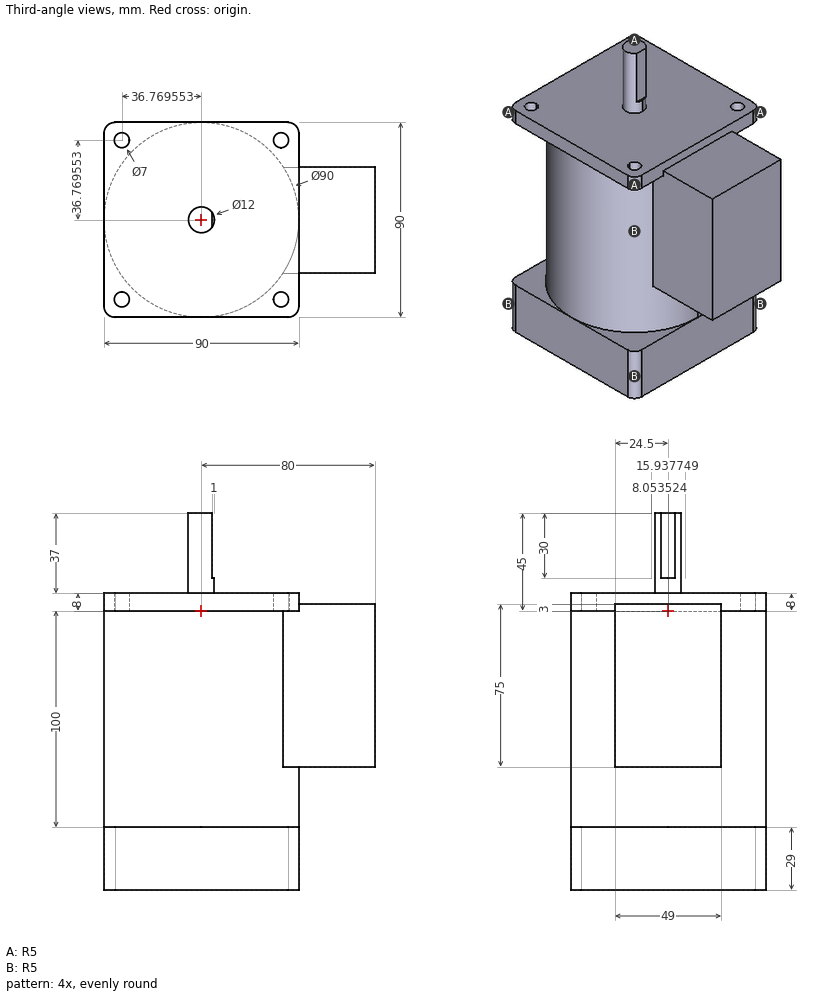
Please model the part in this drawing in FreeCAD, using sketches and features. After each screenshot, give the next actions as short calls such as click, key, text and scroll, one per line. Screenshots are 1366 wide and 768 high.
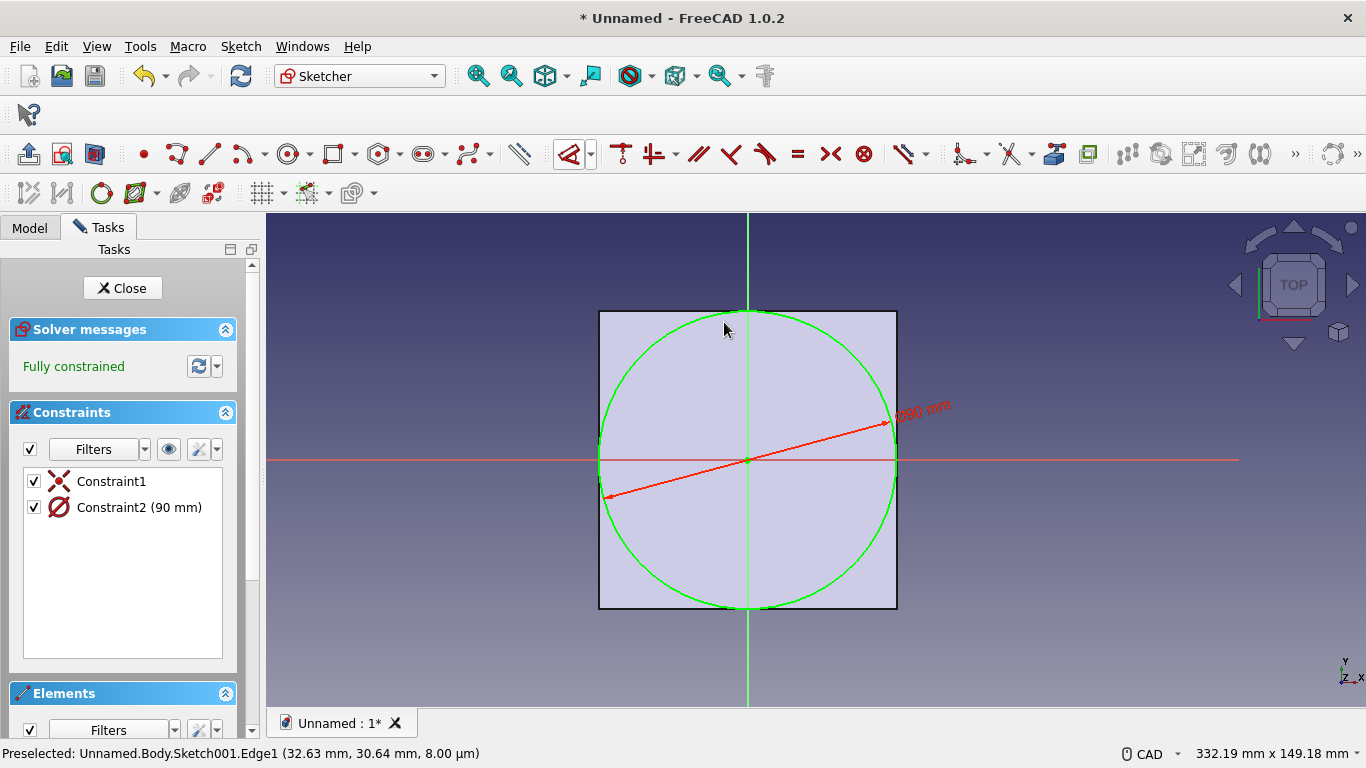
click(123, 288)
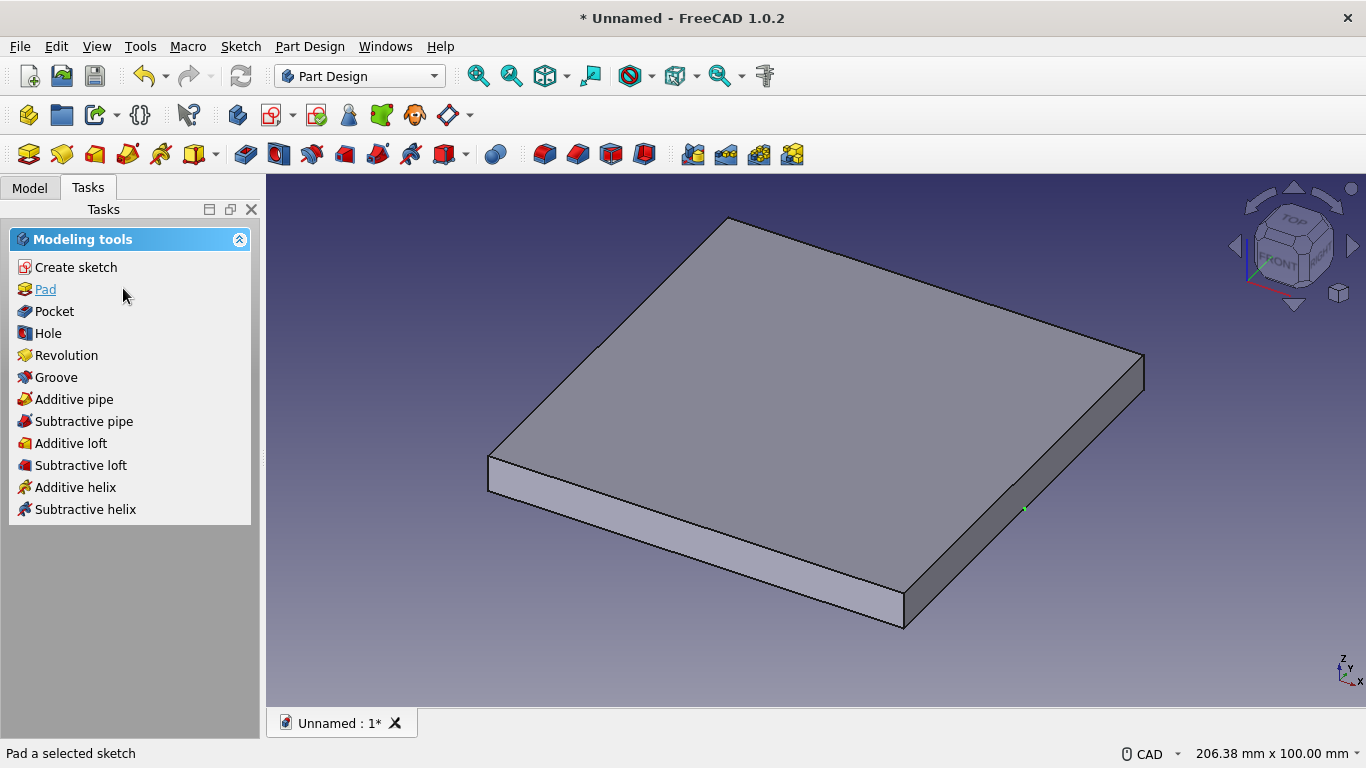
click(29, 154)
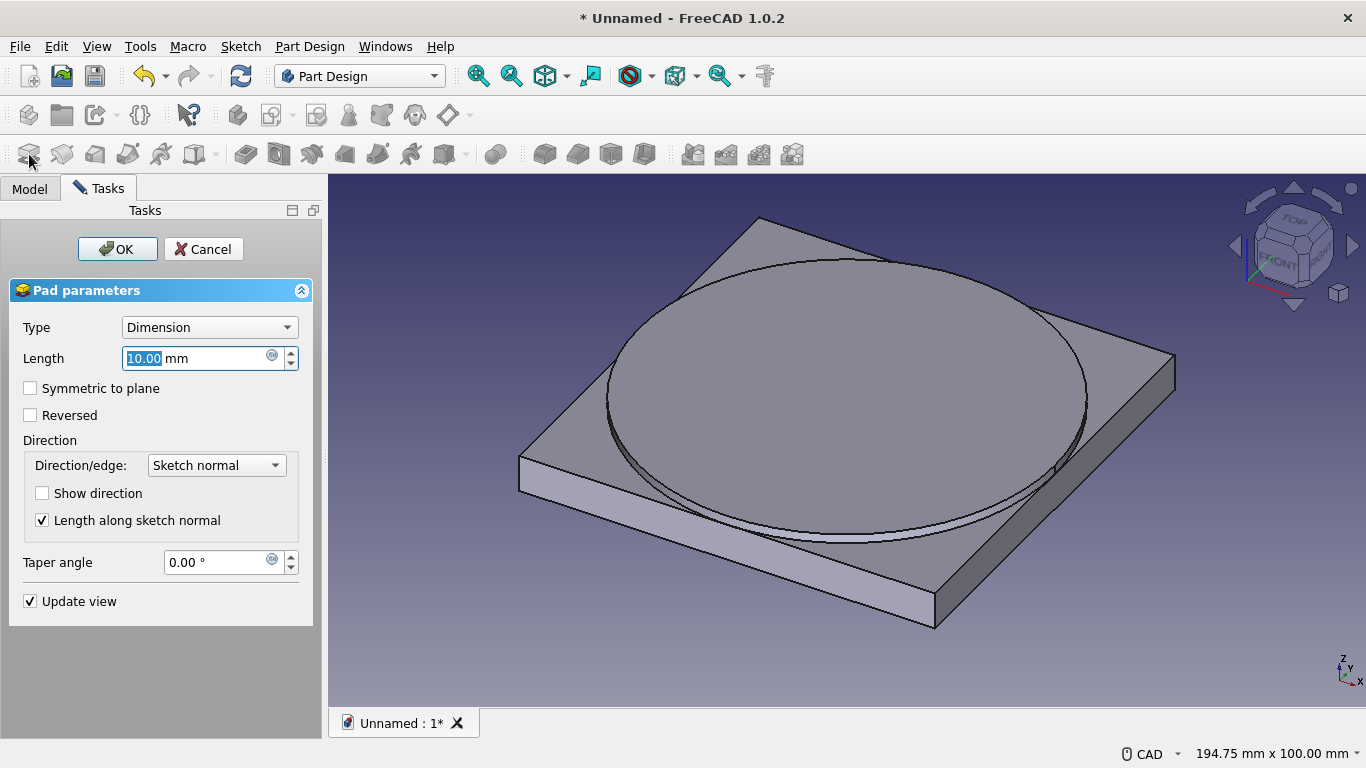
text(100)
key(Tab)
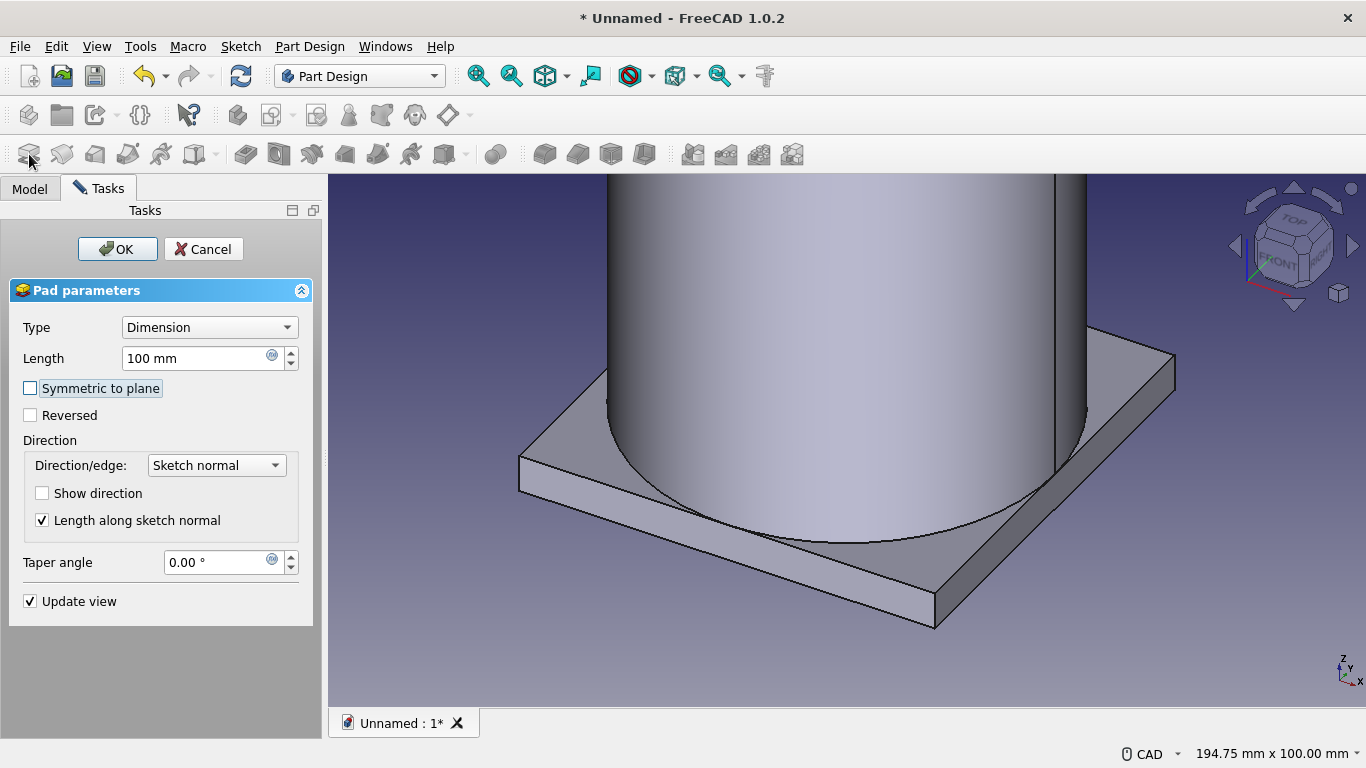
click(31, 415)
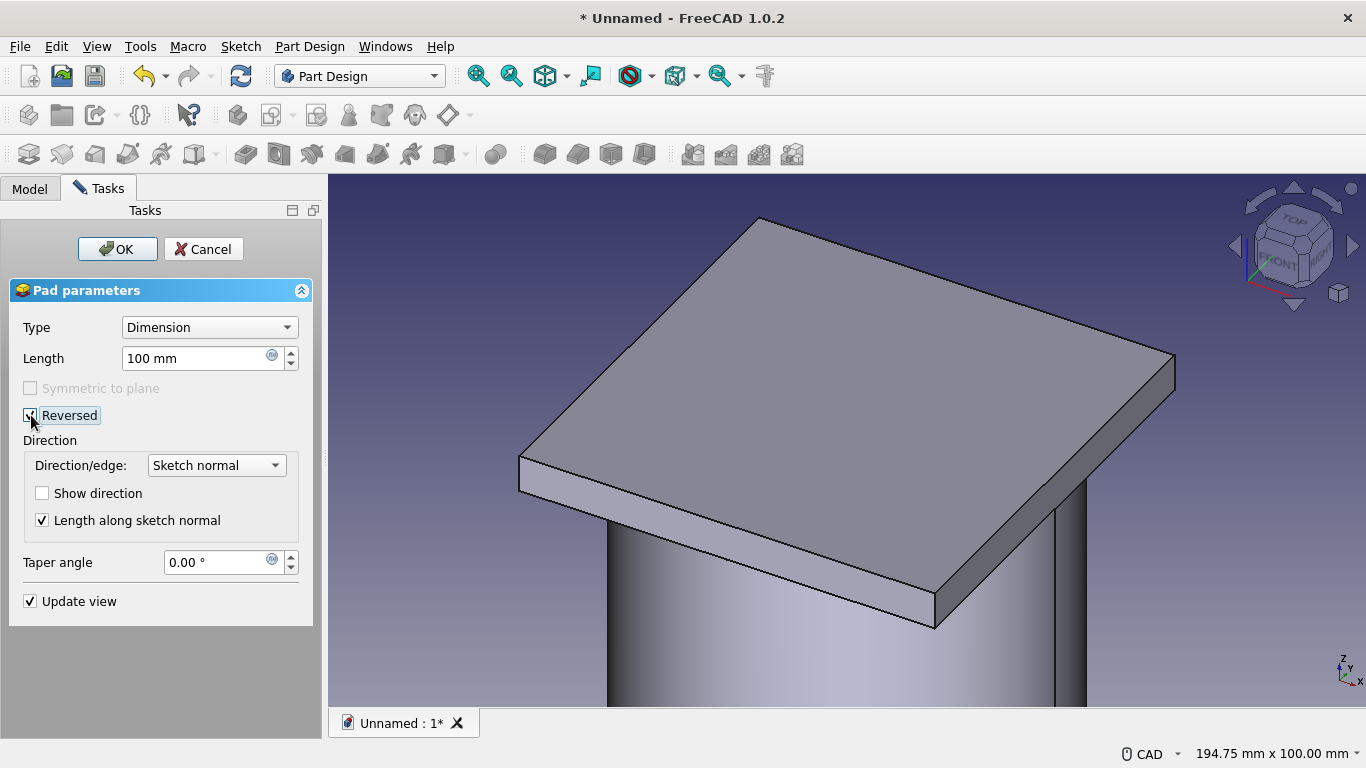
click(118, 249)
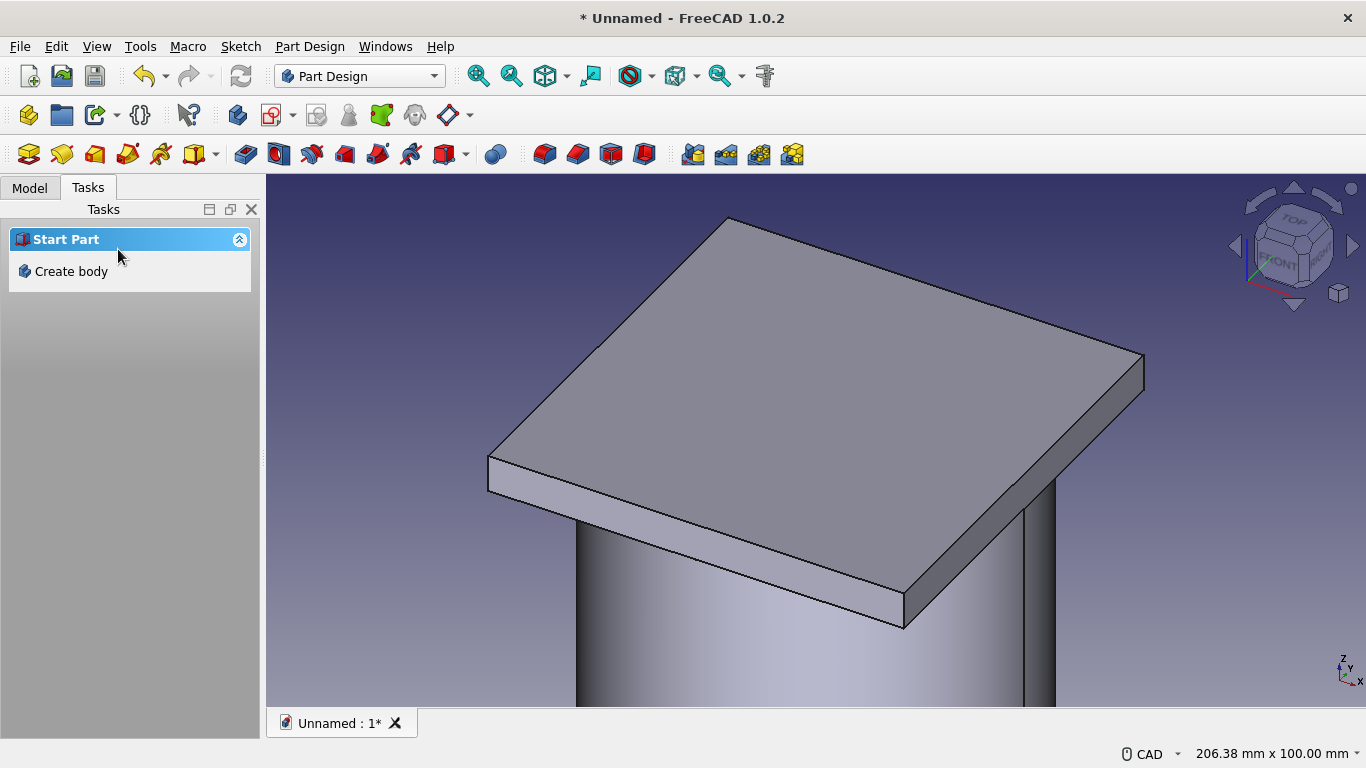
click(479, 76)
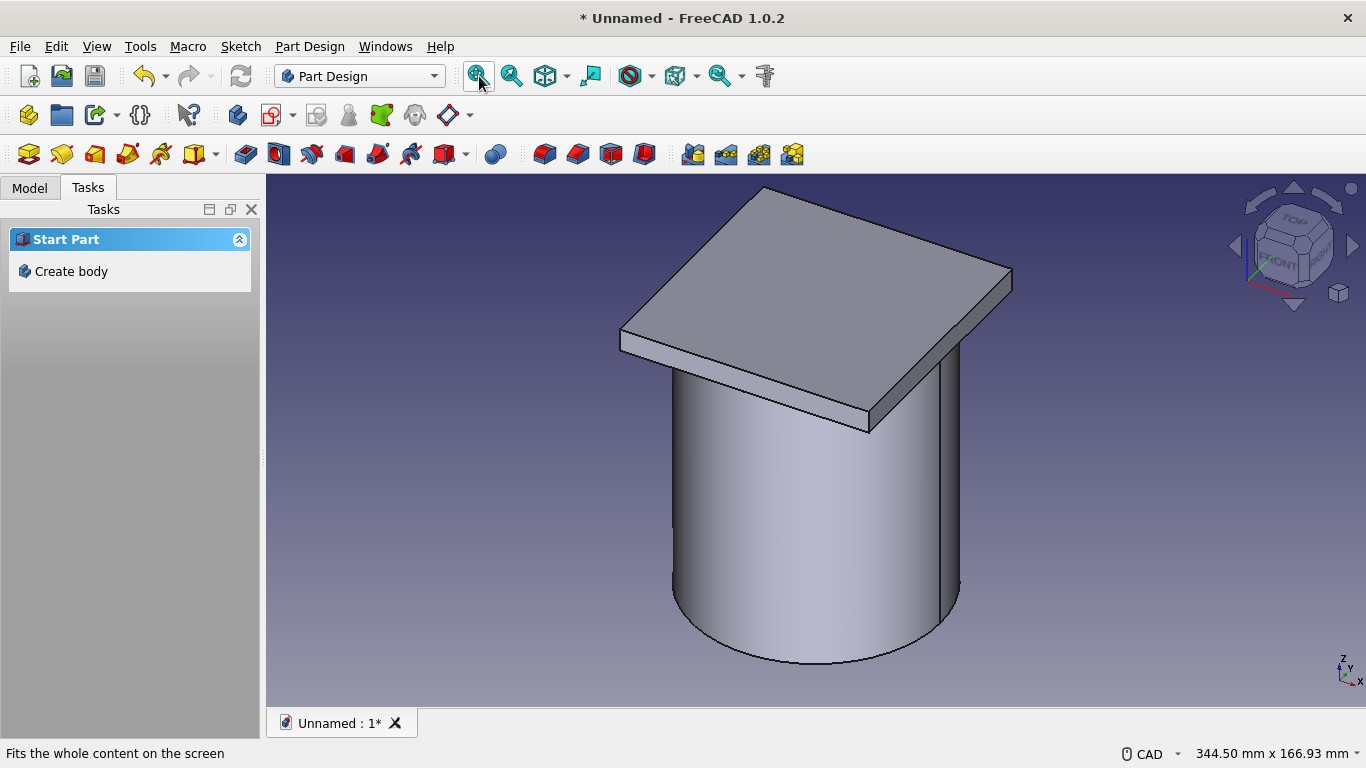
key(5)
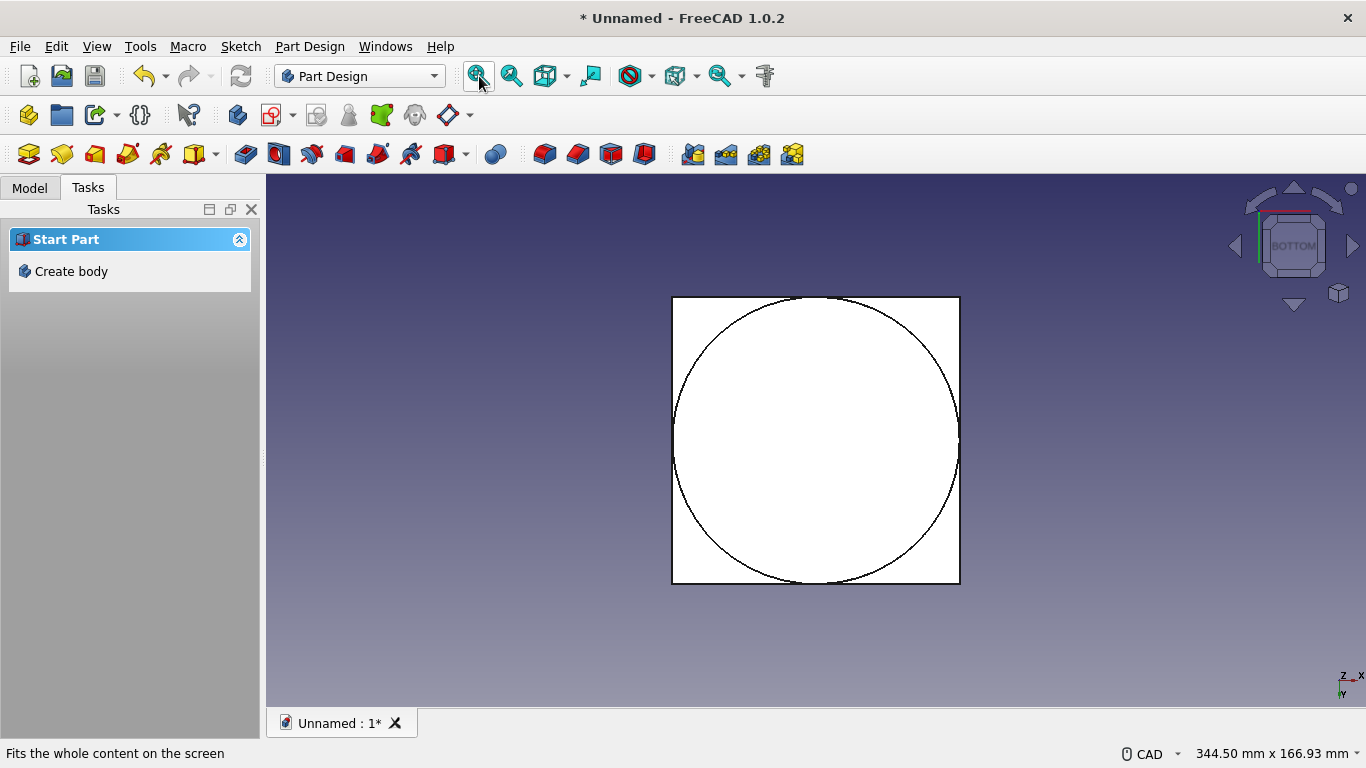
click(816, 439)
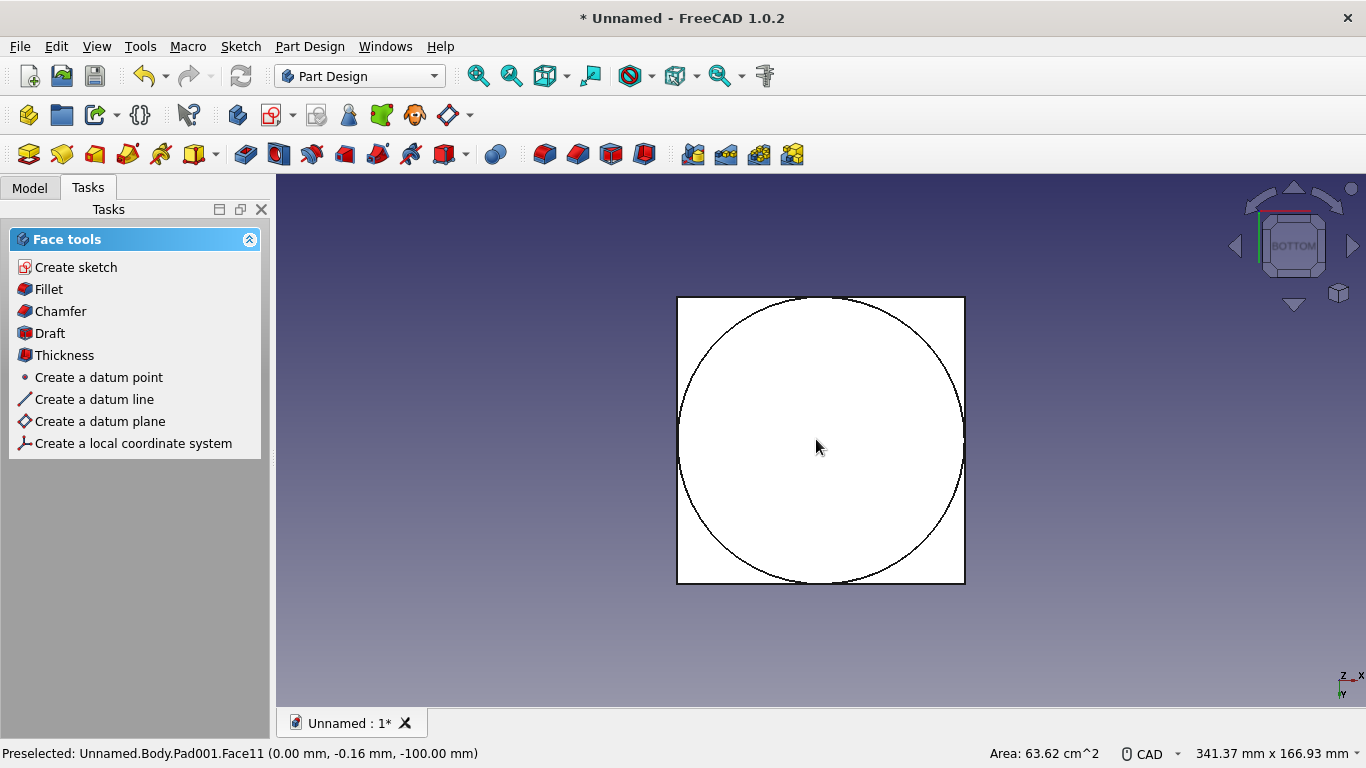
click(270, 116)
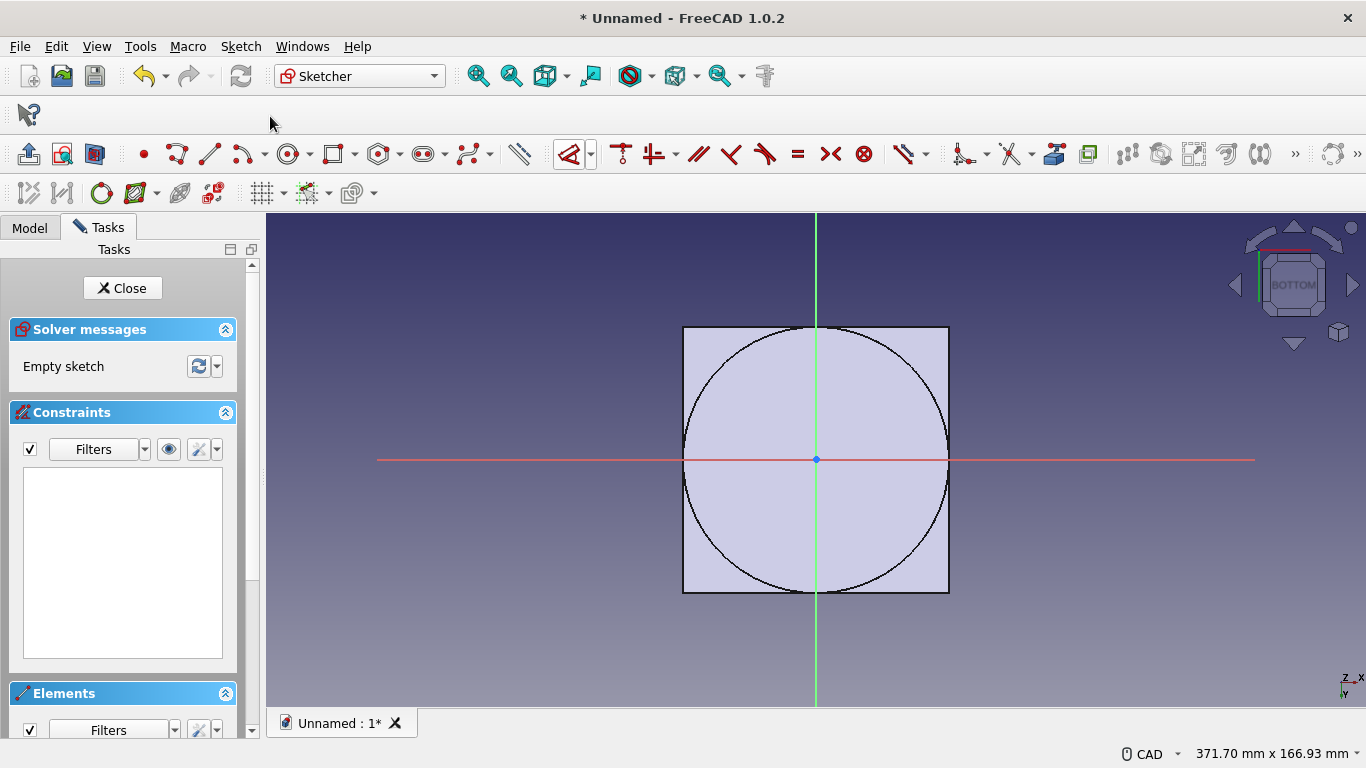
click(354, 154)